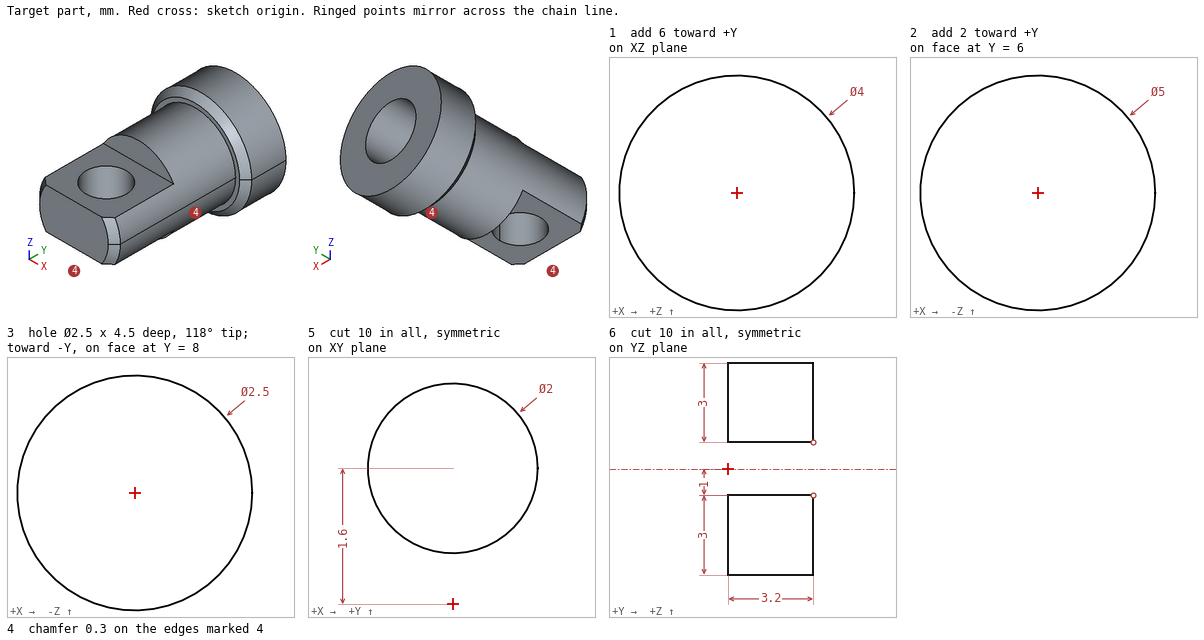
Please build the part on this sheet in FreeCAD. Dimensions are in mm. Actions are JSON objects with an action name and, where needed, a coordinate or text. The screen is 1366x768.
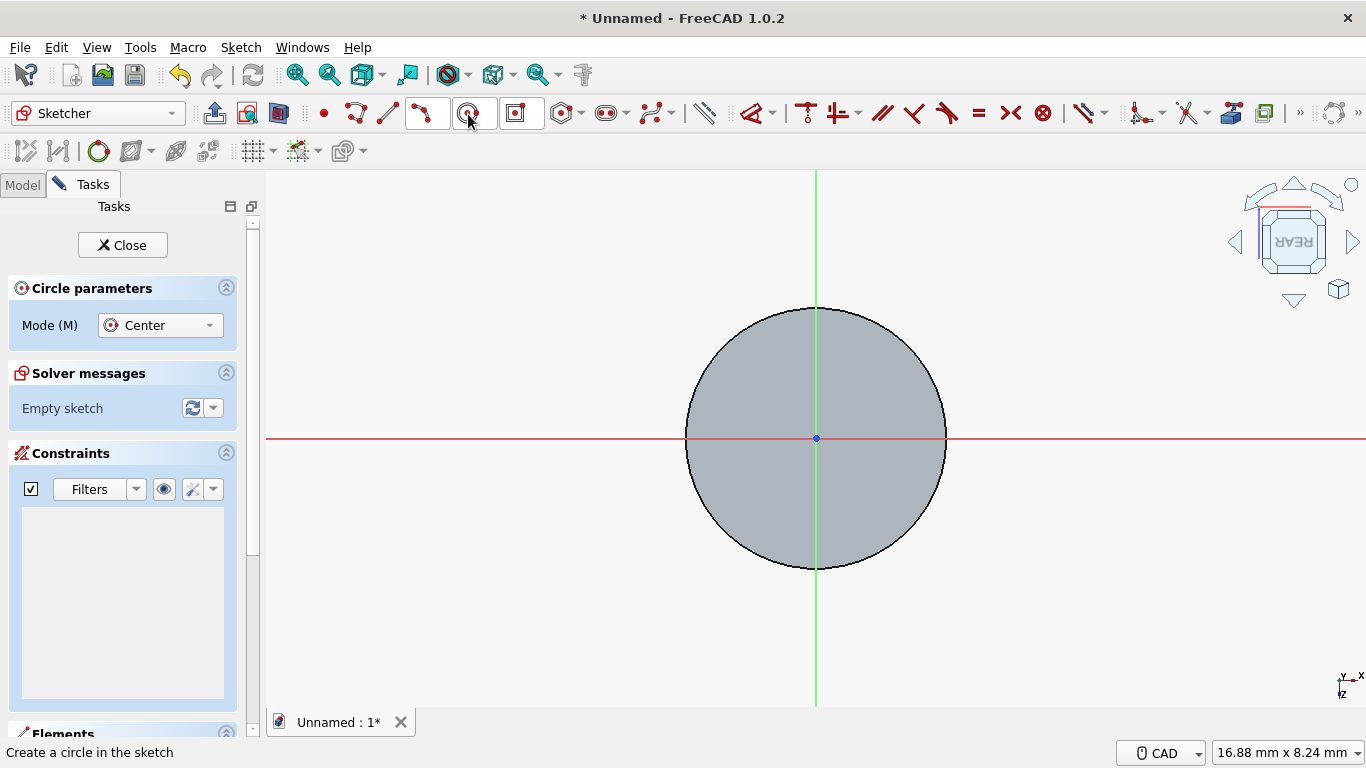
{"action": "left_click", "coordinate": [816, 438]}
{"action": "left_click", "coordinate": [931, 323]}
{"action": "key", "text": "Escape"}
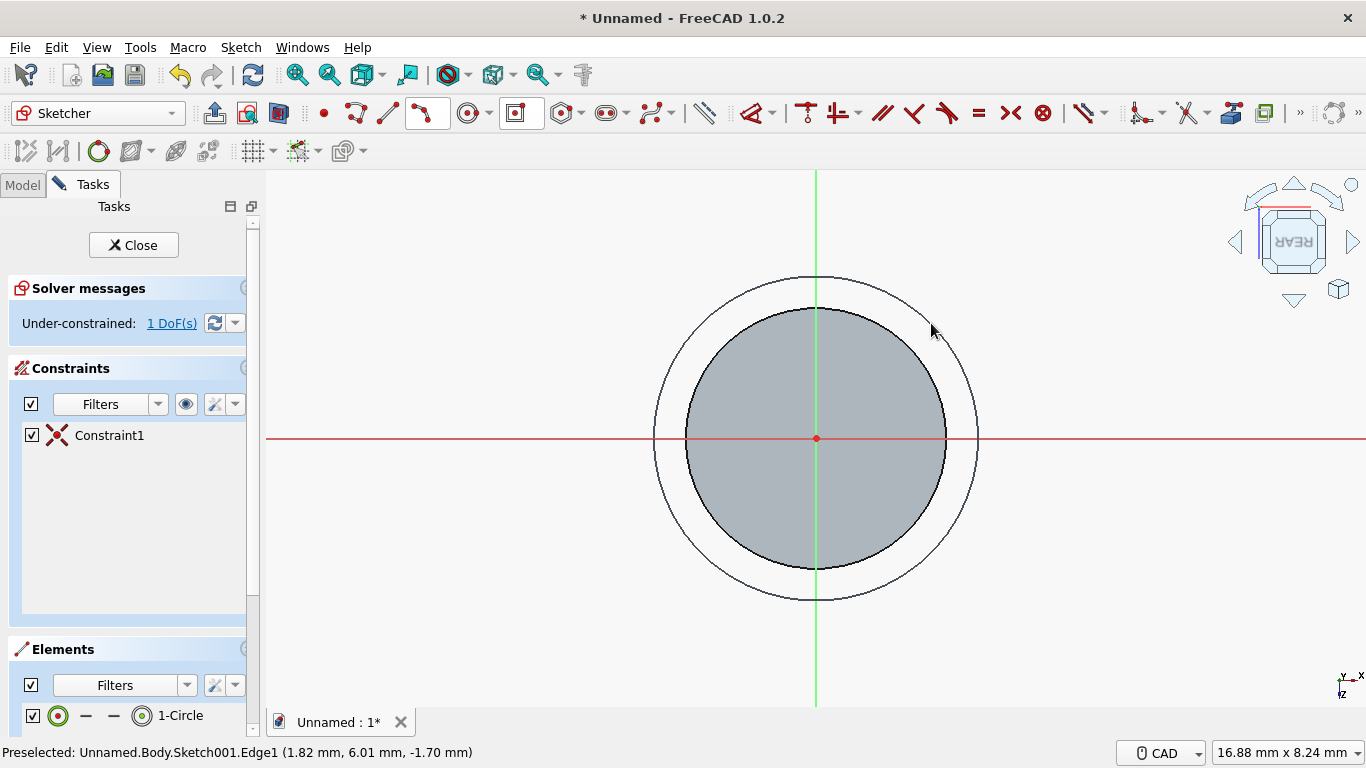
{"action": "left_click", "coordinate": [930, 323]}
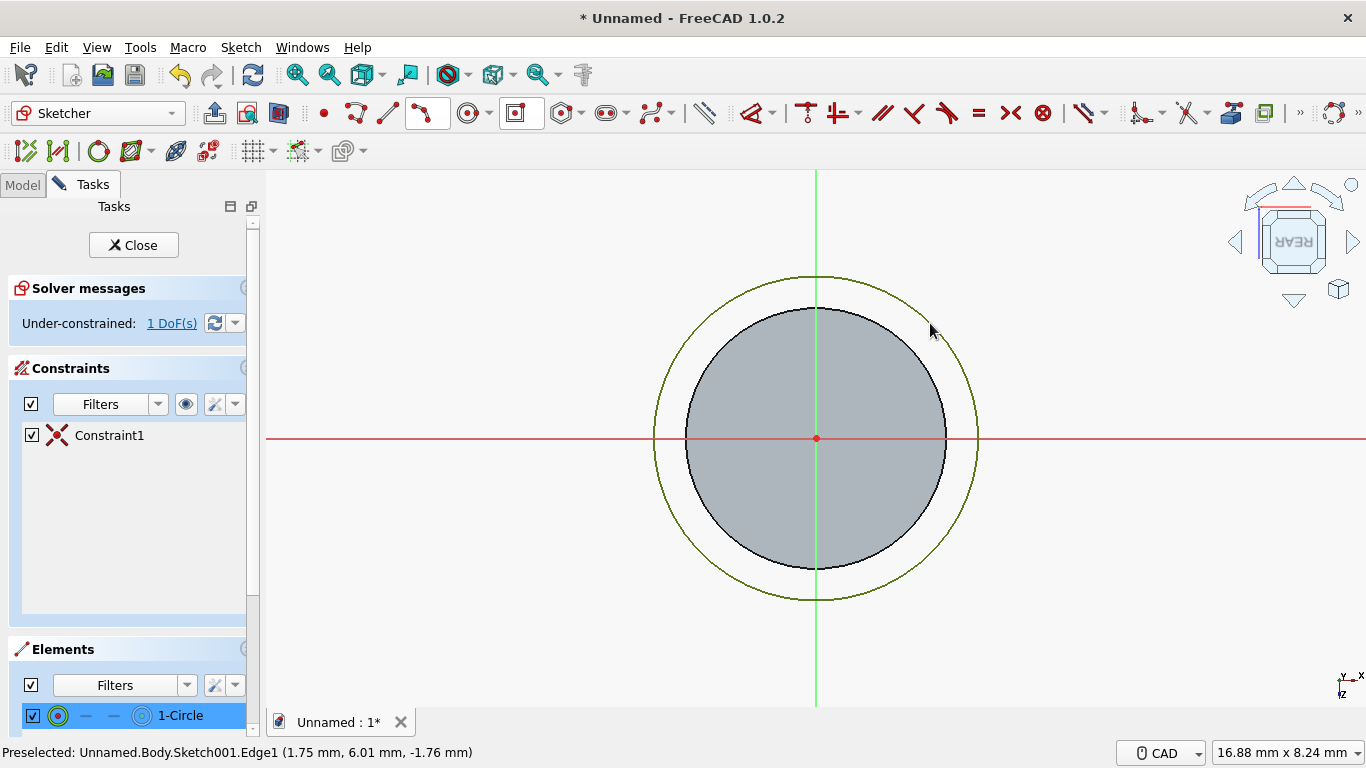
{"action": "key", "text": "k o"}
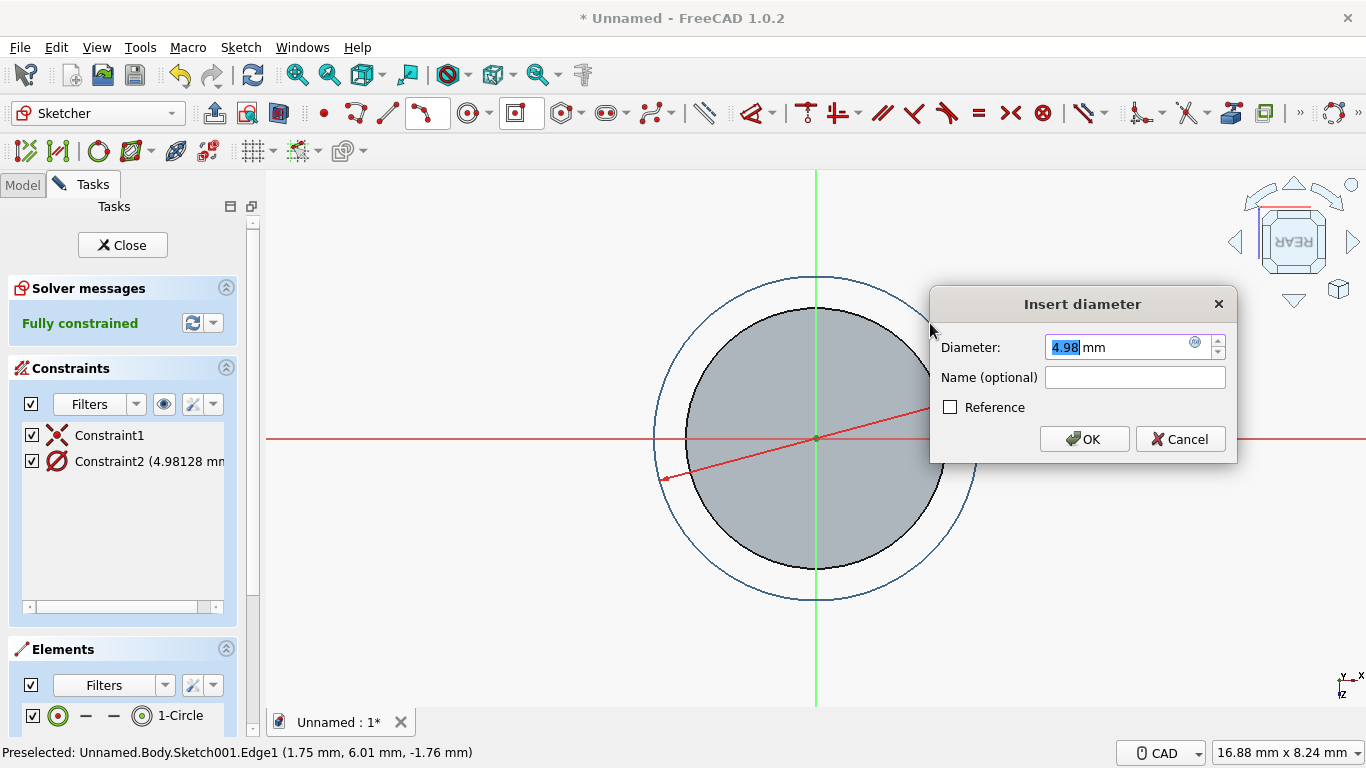
{"action": "type", "text": "5"}
{"action": "key", "text": "Return"}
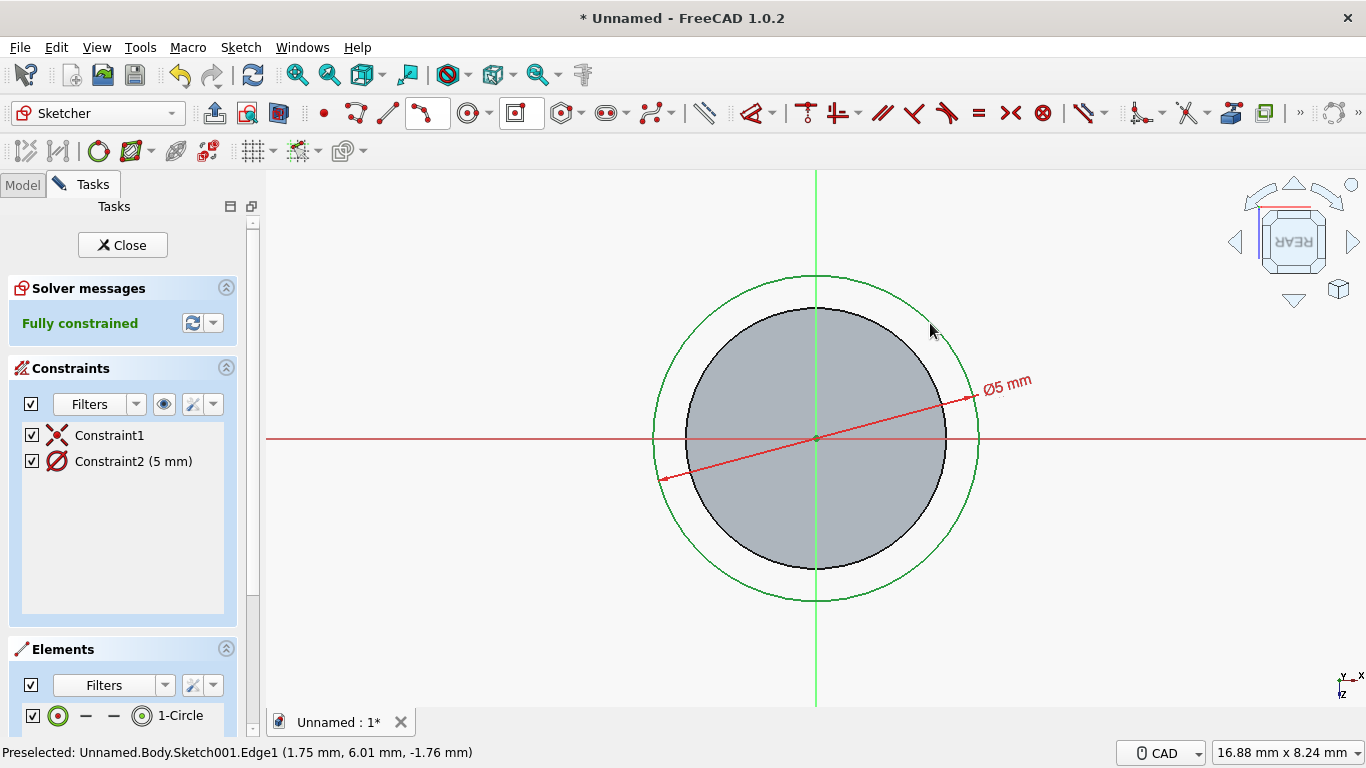
{"action": "left_click", "coordinate": [123, 245]}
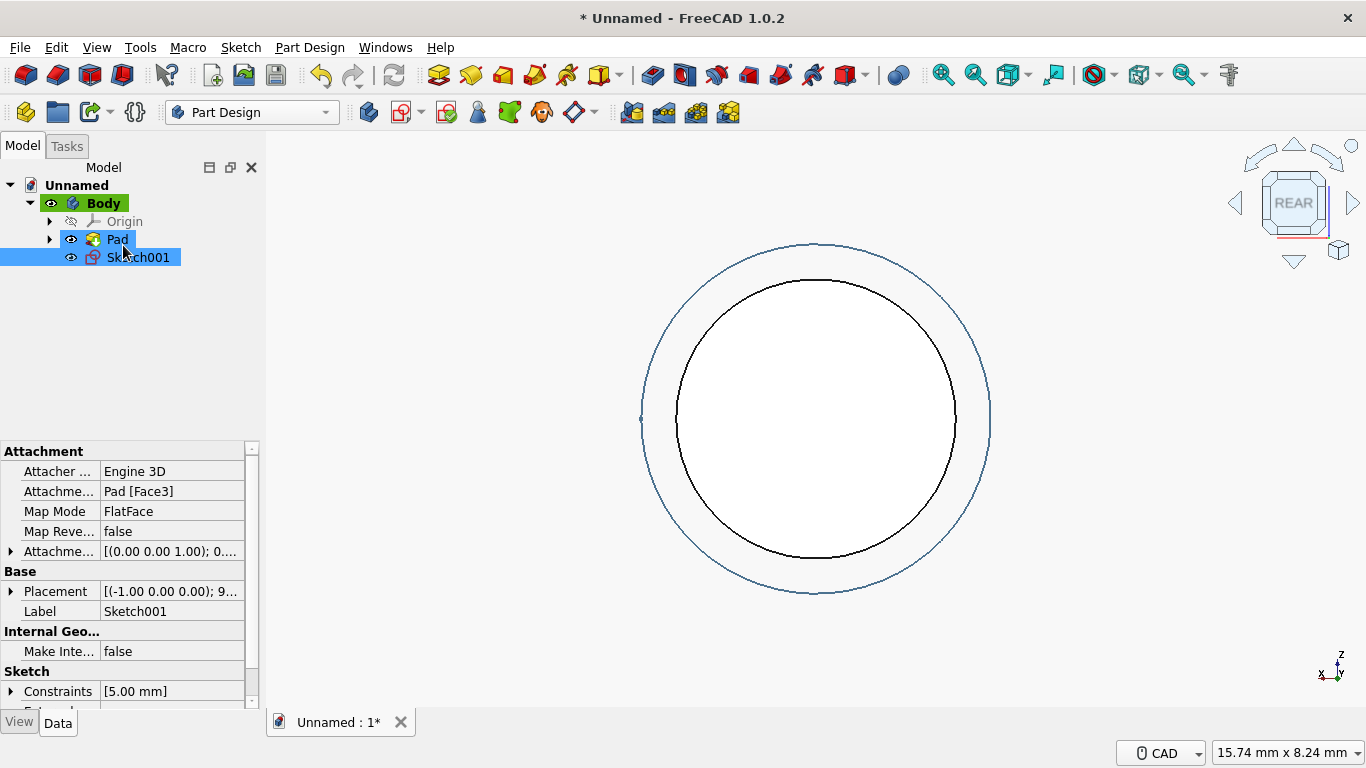
{"action": "left_click", "coordinate": [440, 76]}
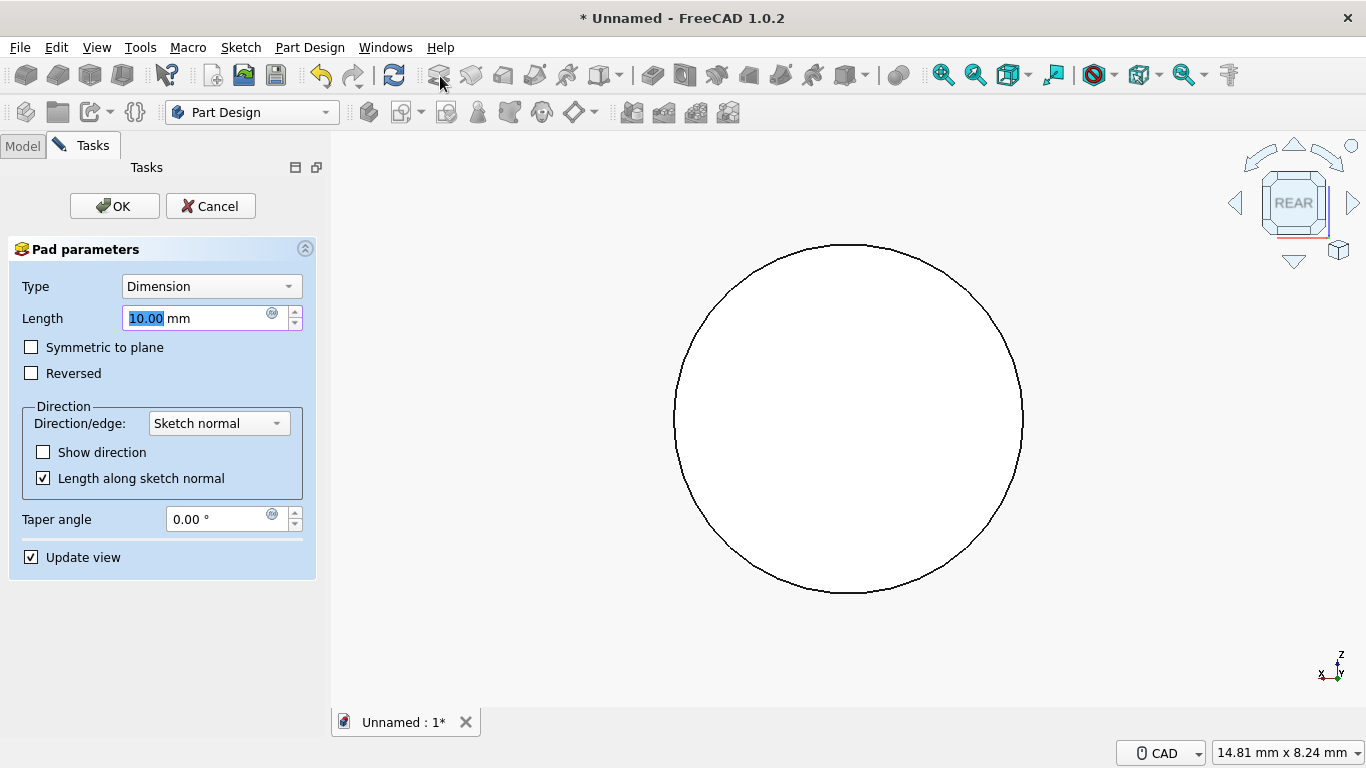
{"action": "type", "text": "2"}
{"action": "key", "text": "Tab"}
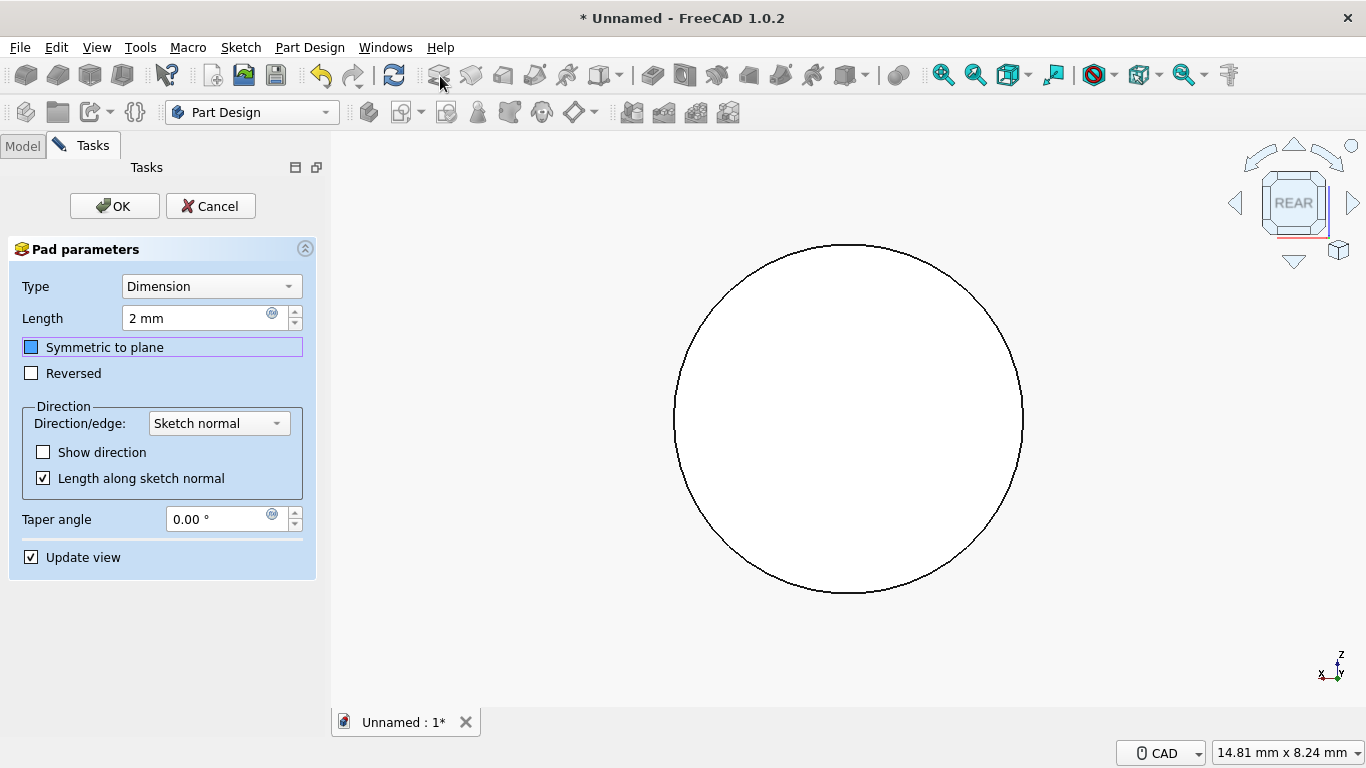
{"action": "left_click", "coordinate": [115, 206]}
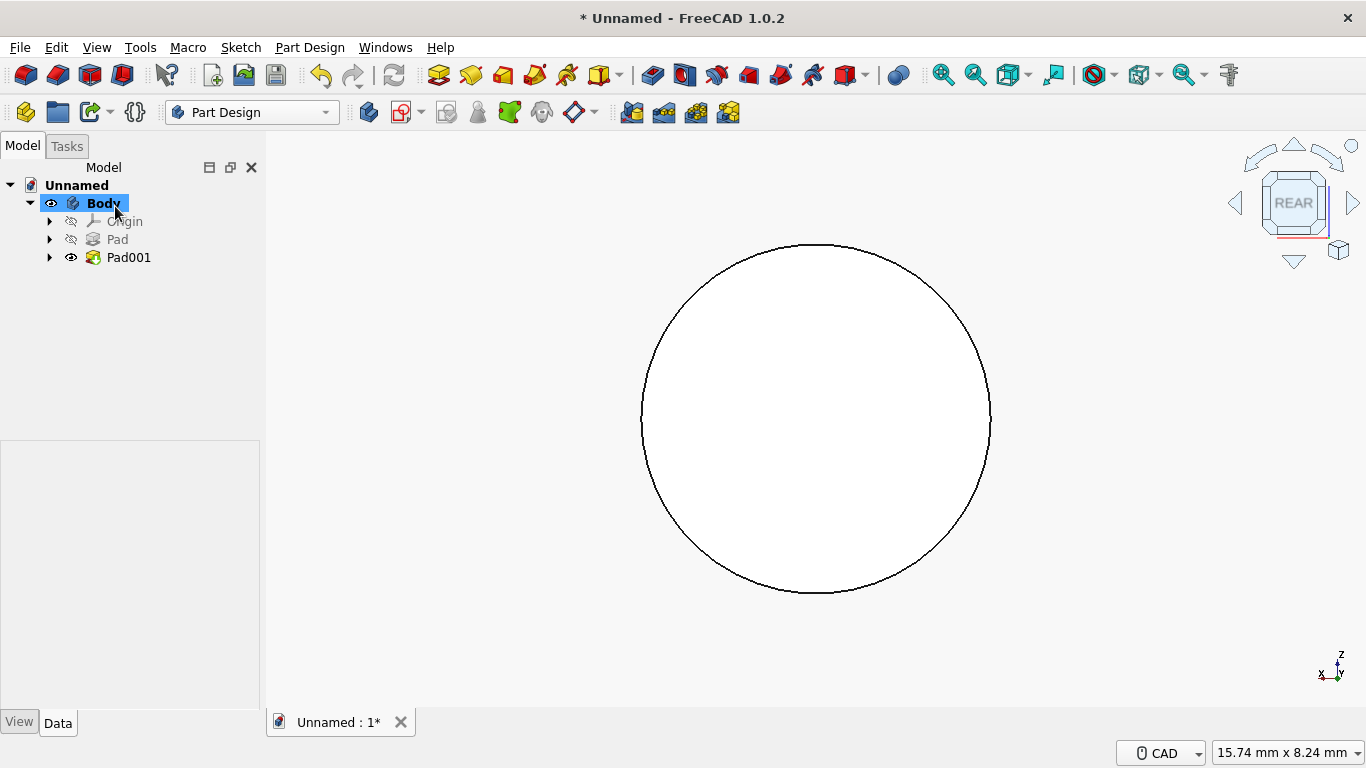
{"action": "left_click", "coordinate": [816, 418]}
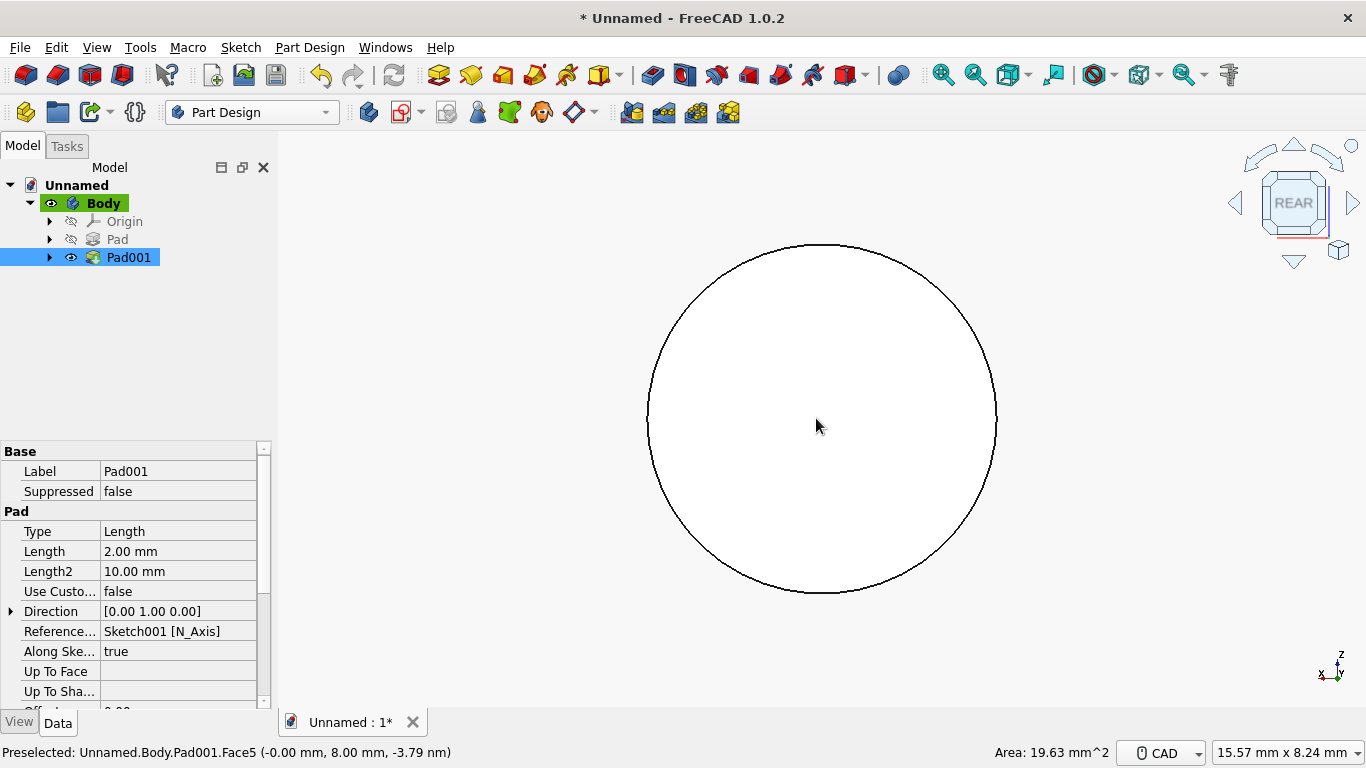
{"action": "left_click", "coordinate": [402, 112]}